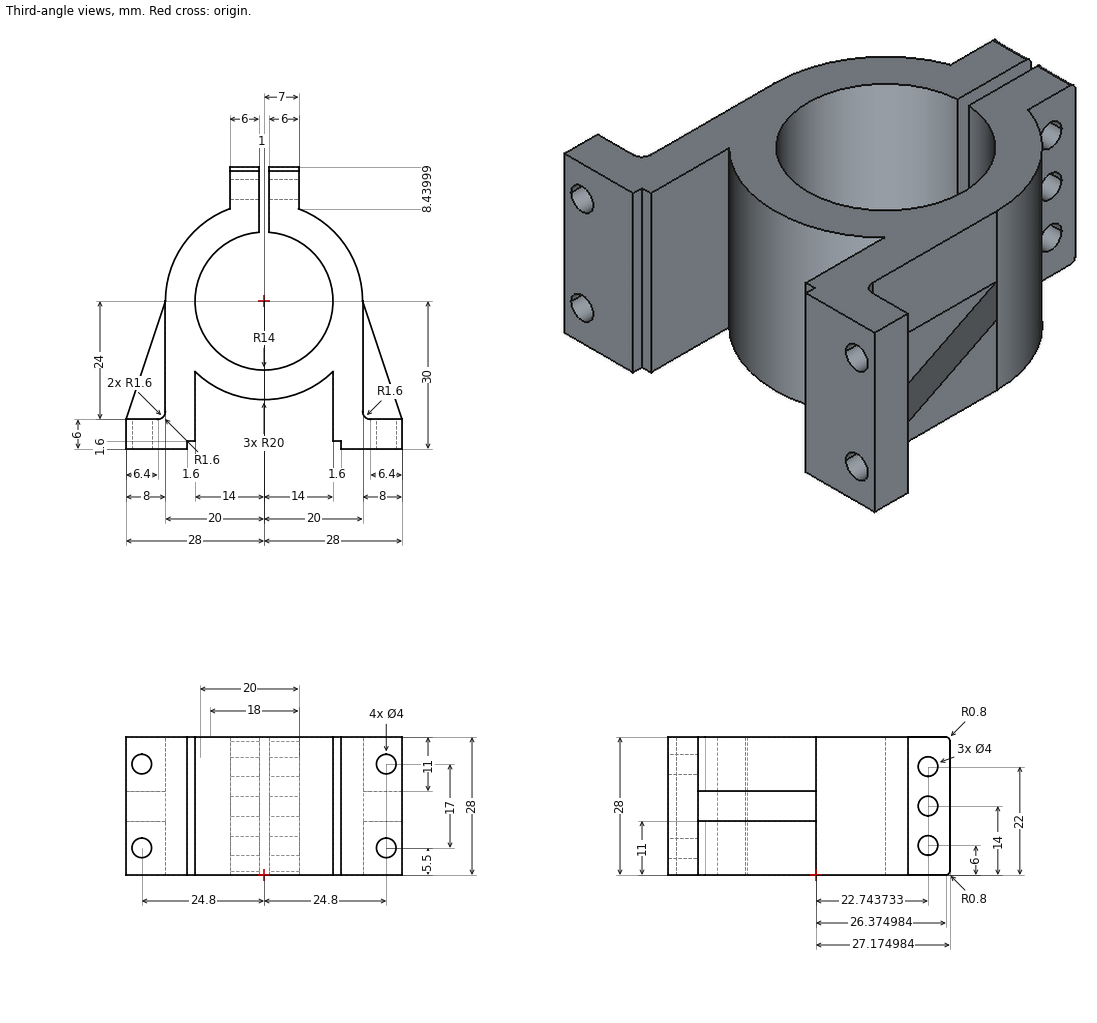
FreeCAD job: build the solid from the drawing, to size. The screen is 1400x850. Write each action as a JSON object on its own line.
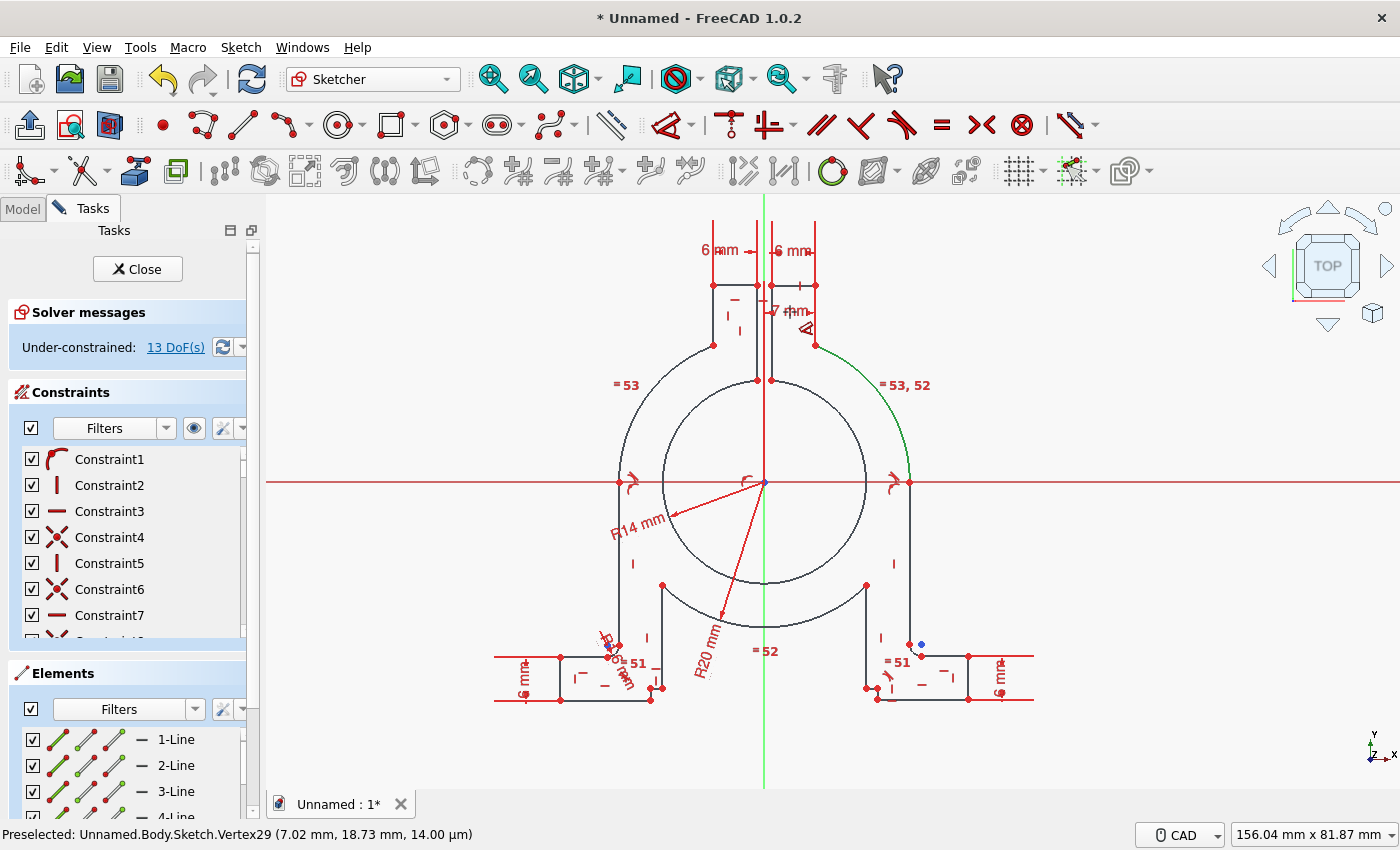
{"action": "scroll", "coordinate": [757, 381], "scroll_direction": "up", "scroll_amount": 9}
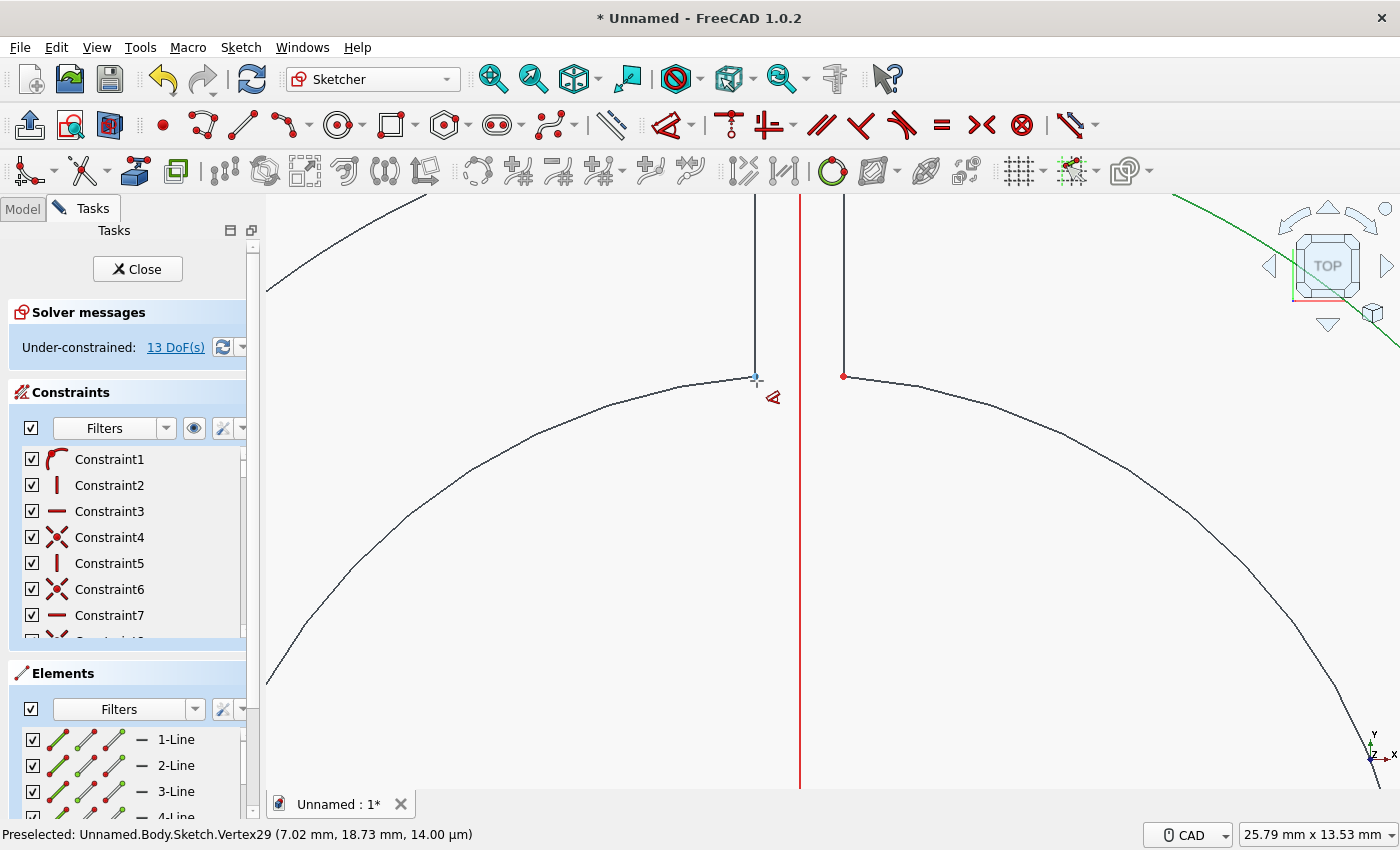
{"action": "left_click", "coordinate": [755, 377]}
{"action": "left_click", "coordinate": [778, 343]}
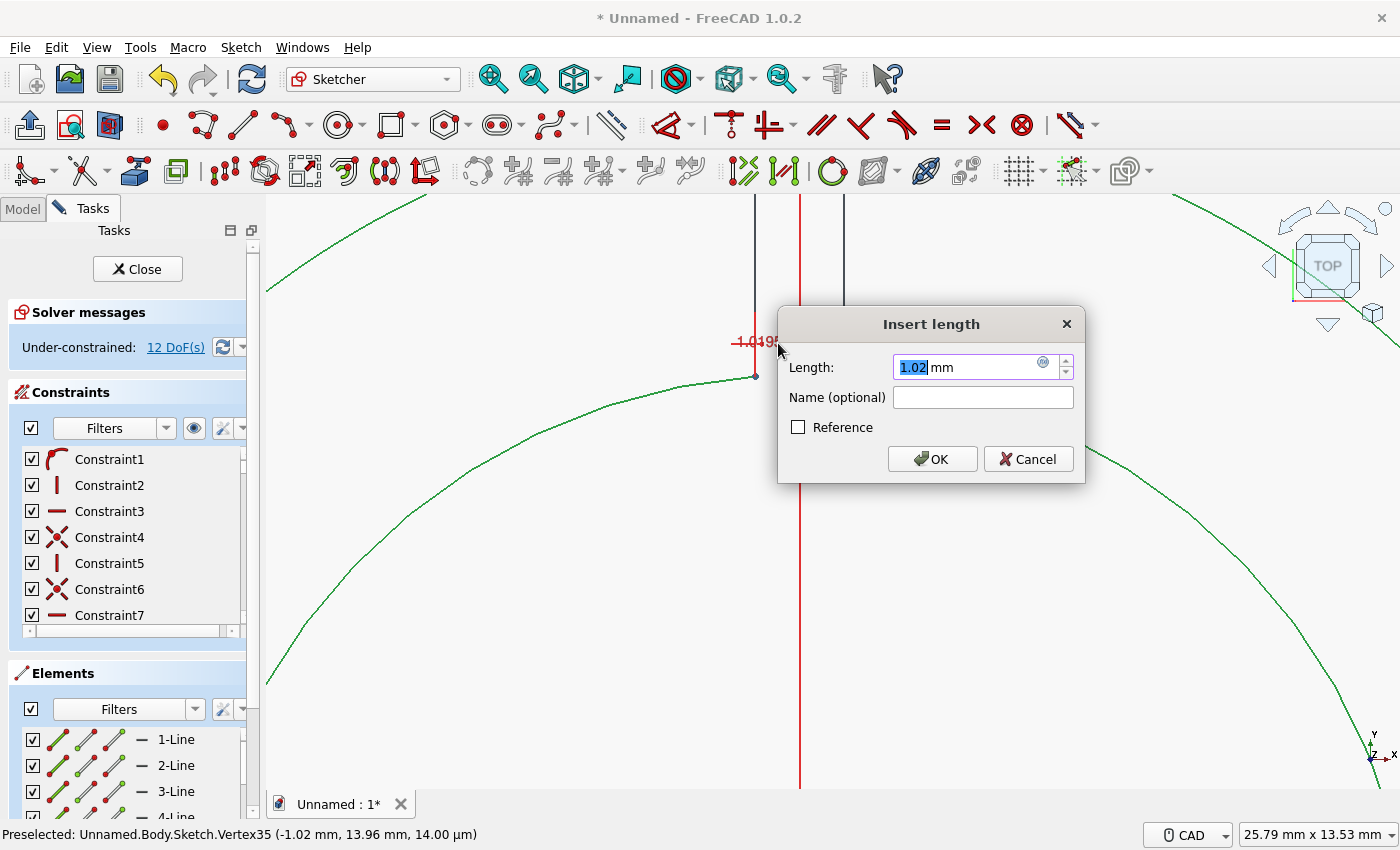
{"action": "type", "text": "1"}
{"action": "key", "text": "Return"}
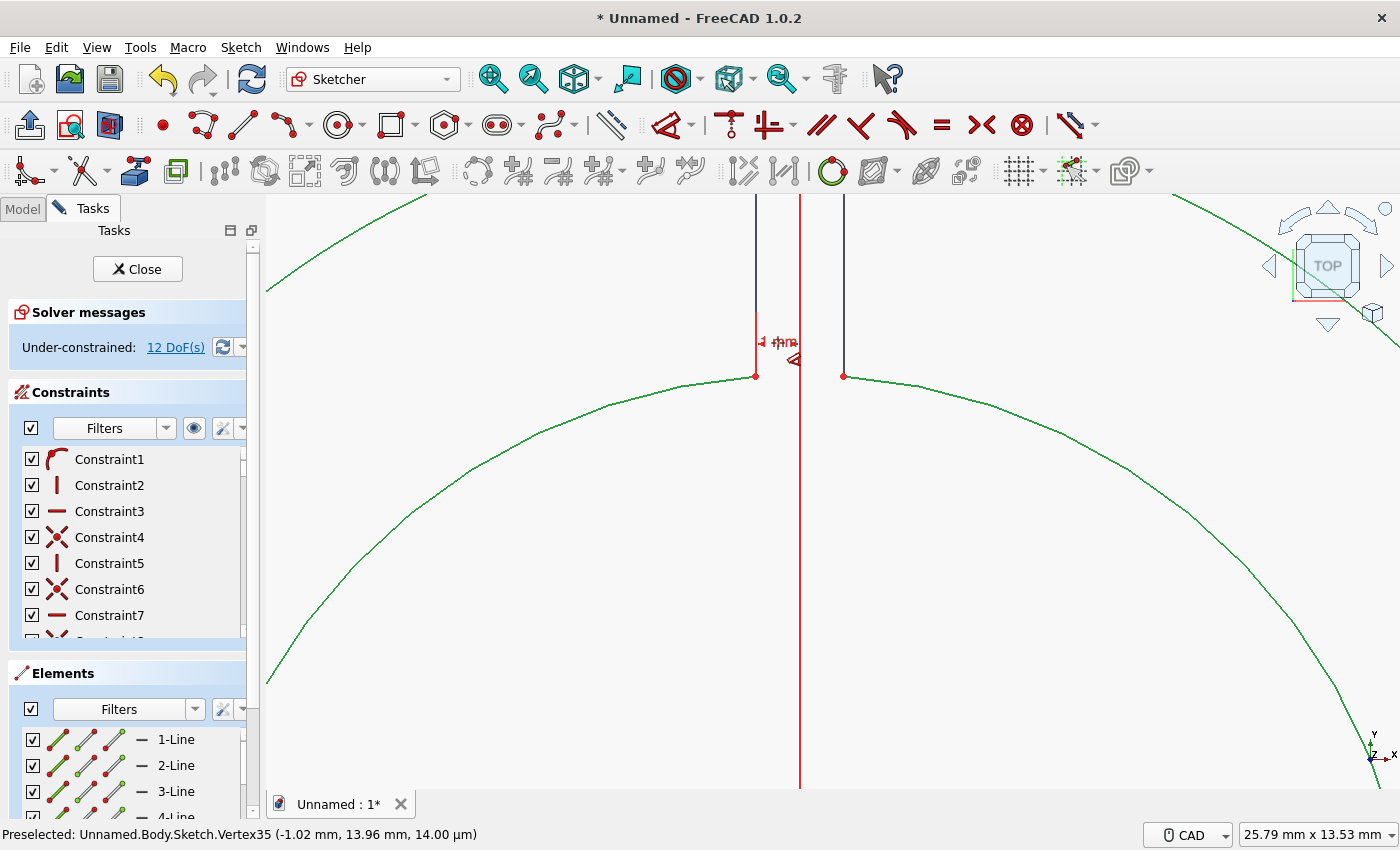
{"action": "scroll", "coordinate": [757, 380], "scroll_direction": "down", "scroll_amount": 9}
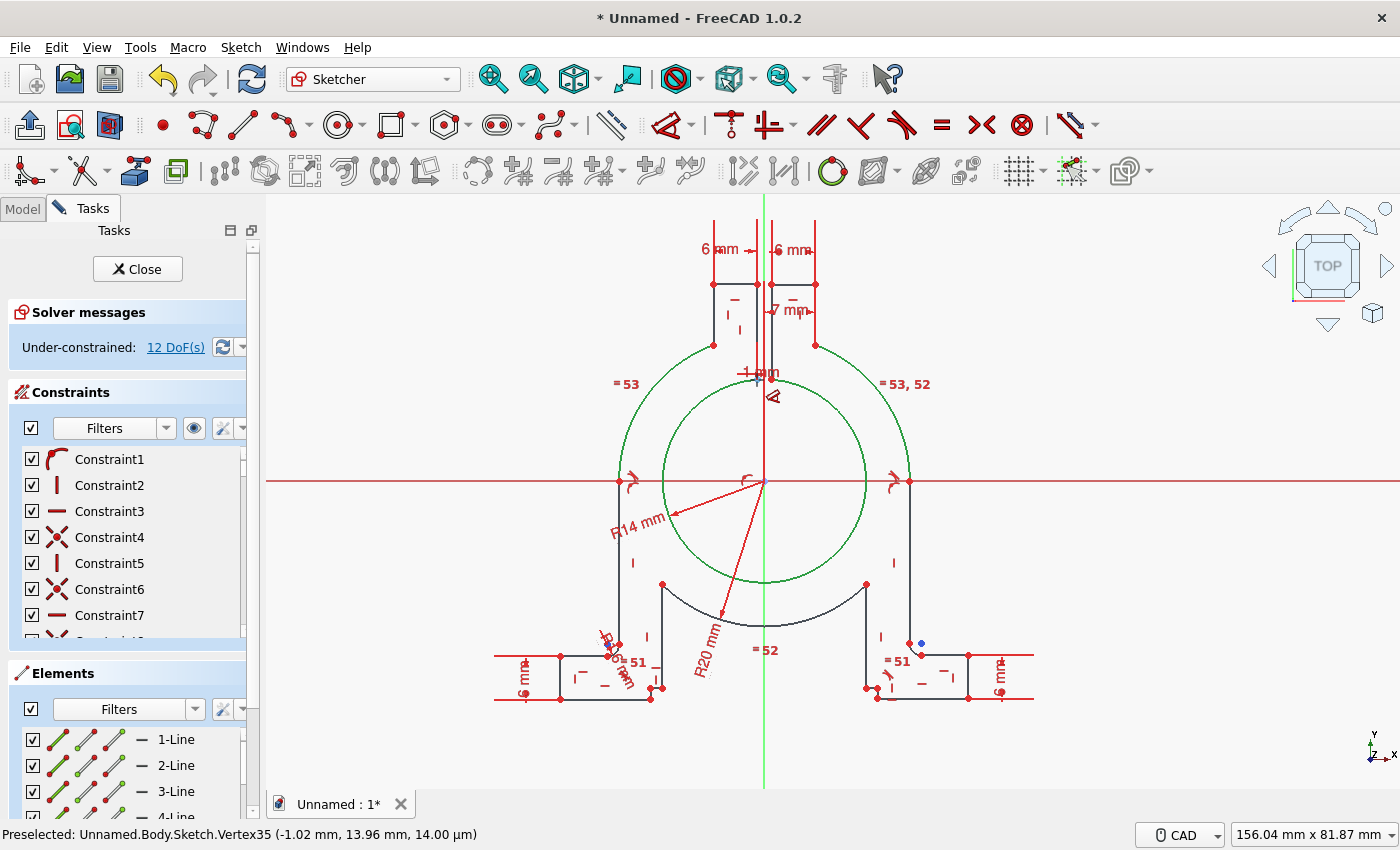
{"action": "left_click", "coordinate": [593, 656]}
{"action": "left_click", "coordinate": [584, 622]}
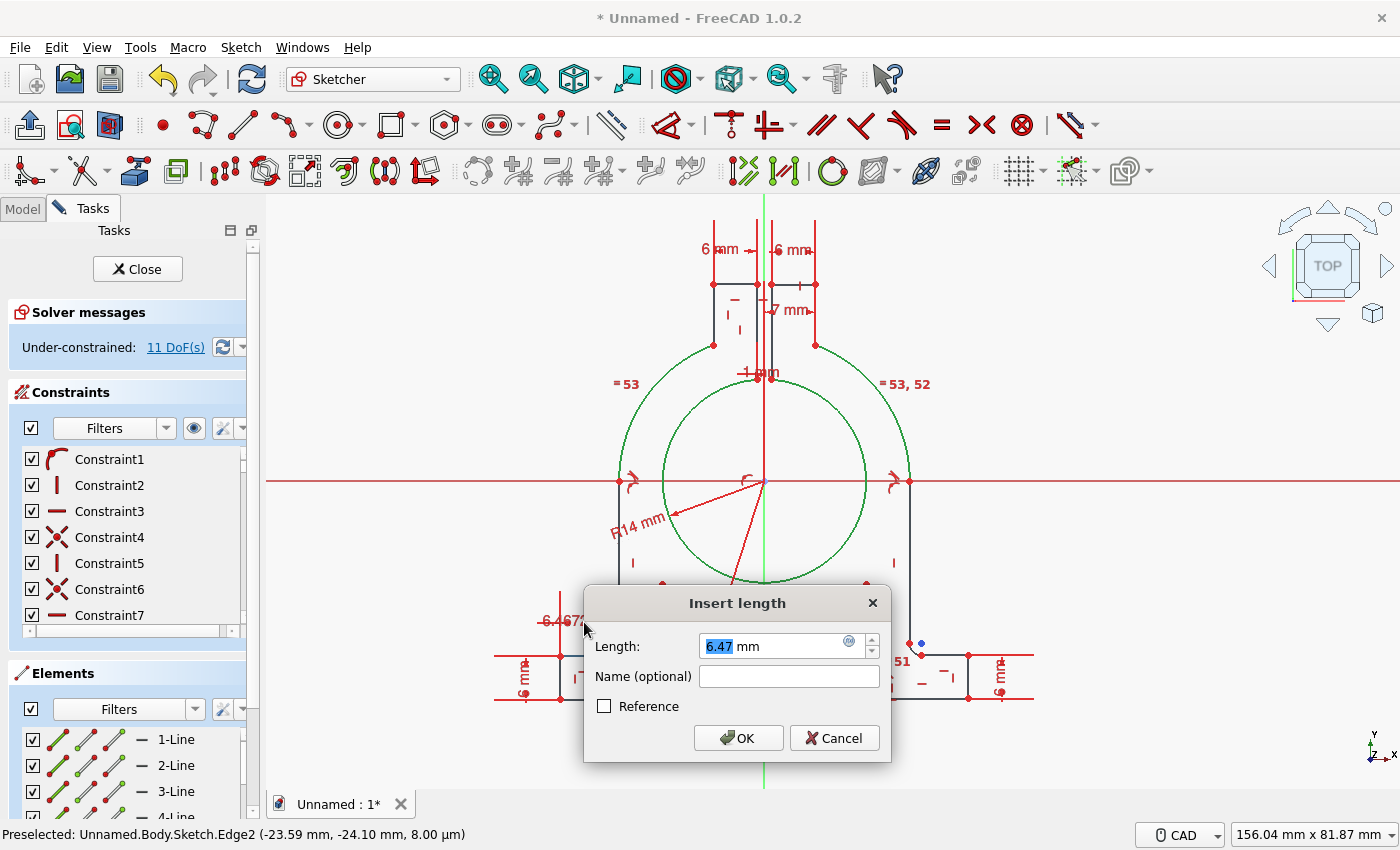
{"action": "type", "text": "6.4"}
{"action": "key", "text": "Return"}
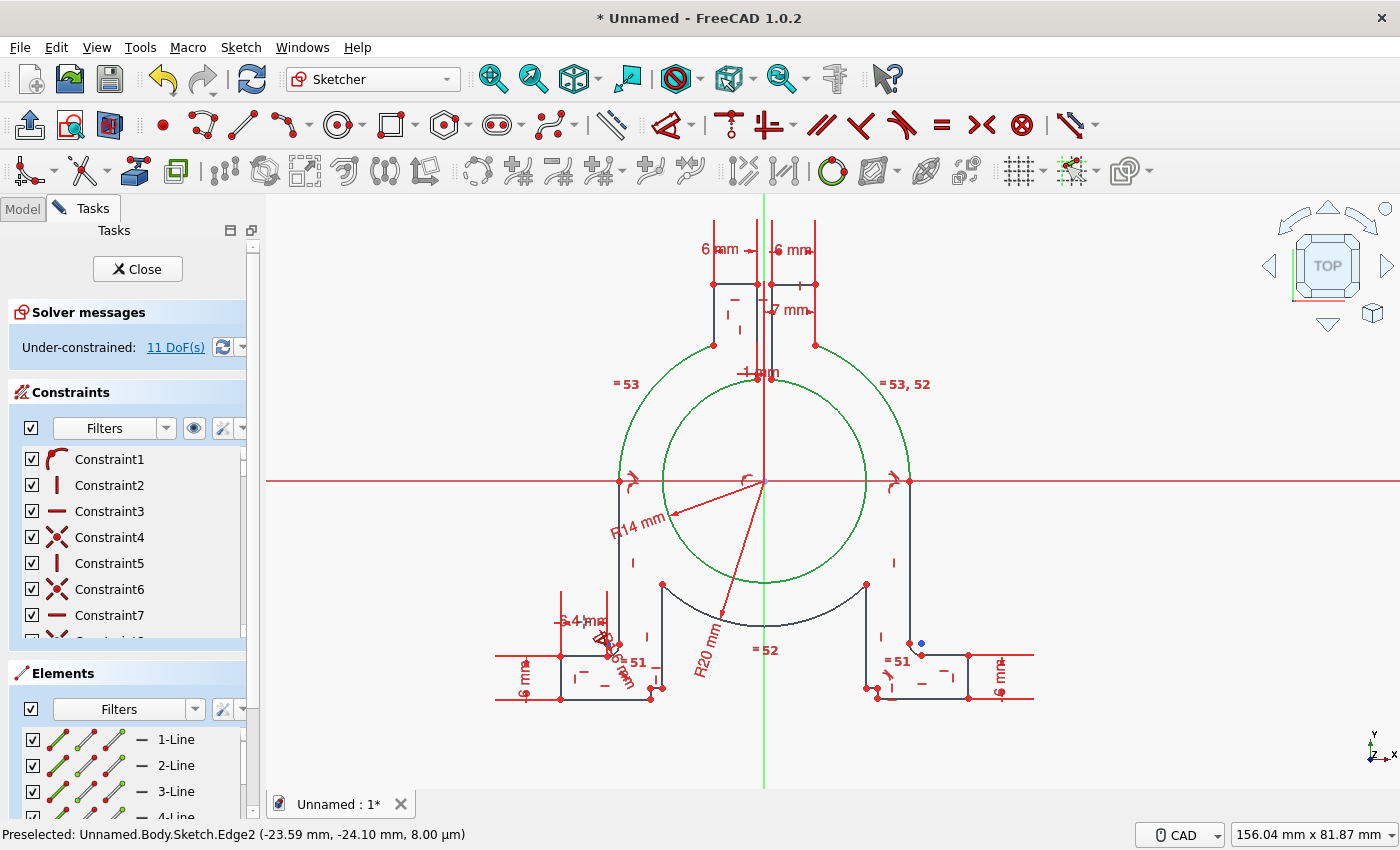
{"action": "scroll", "coordinate": [651, 694], "scroll_direction": "up", "scroll_amount": 7}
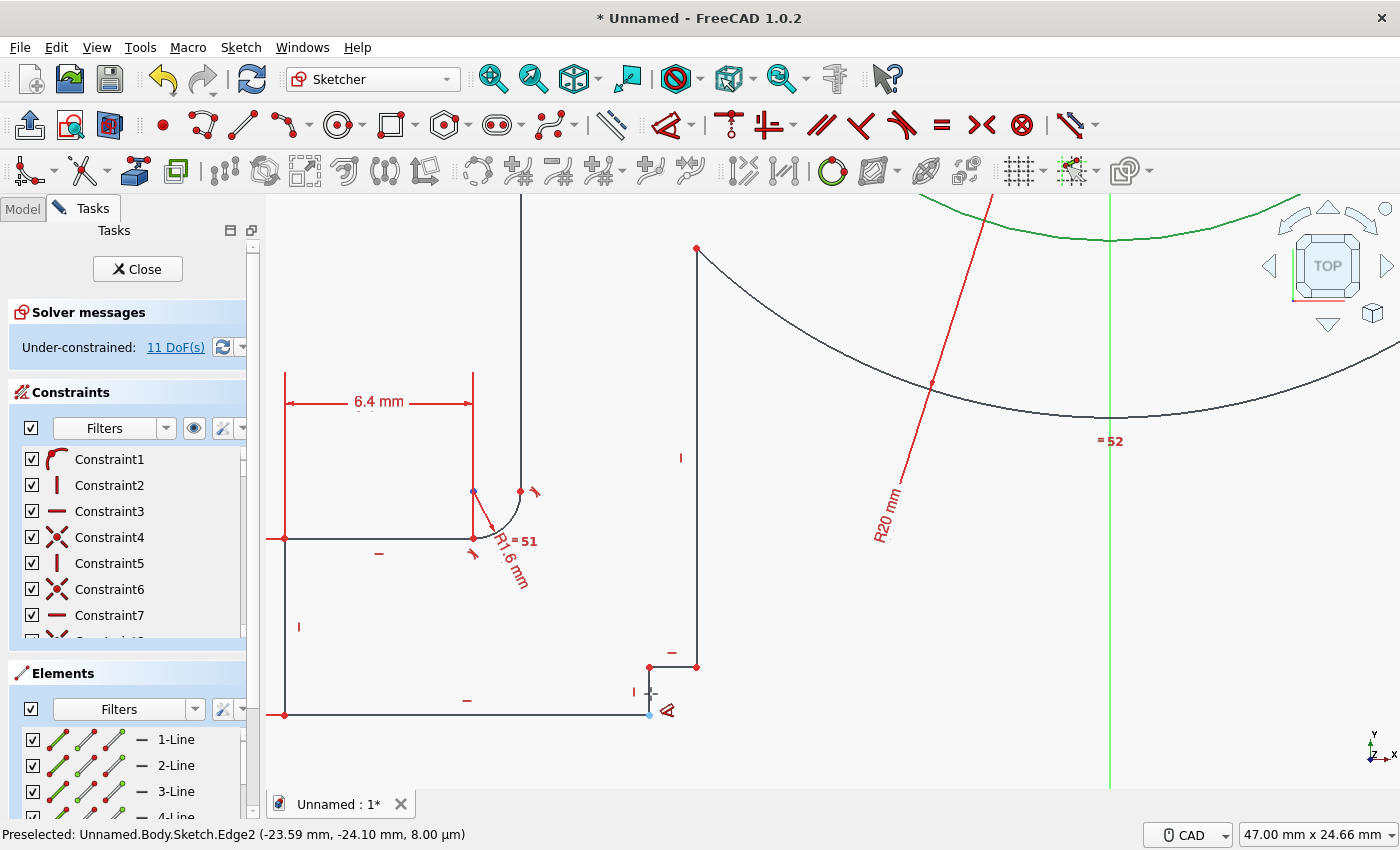
{"action": "left_click", "coordinate": [649, 691]}
{"action": "left_click", "coordinate": [615, 691]}